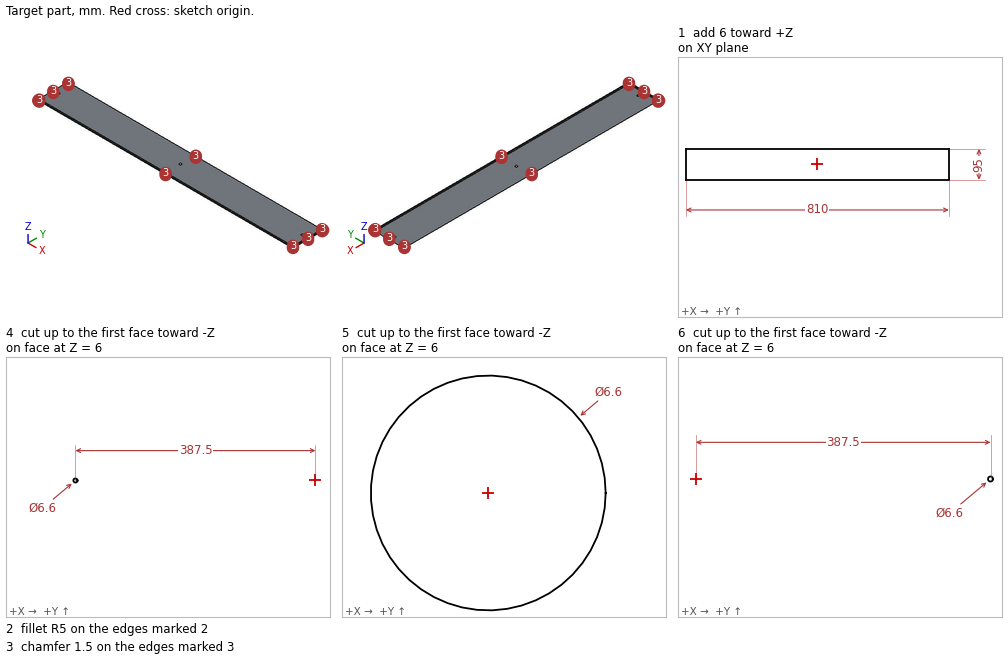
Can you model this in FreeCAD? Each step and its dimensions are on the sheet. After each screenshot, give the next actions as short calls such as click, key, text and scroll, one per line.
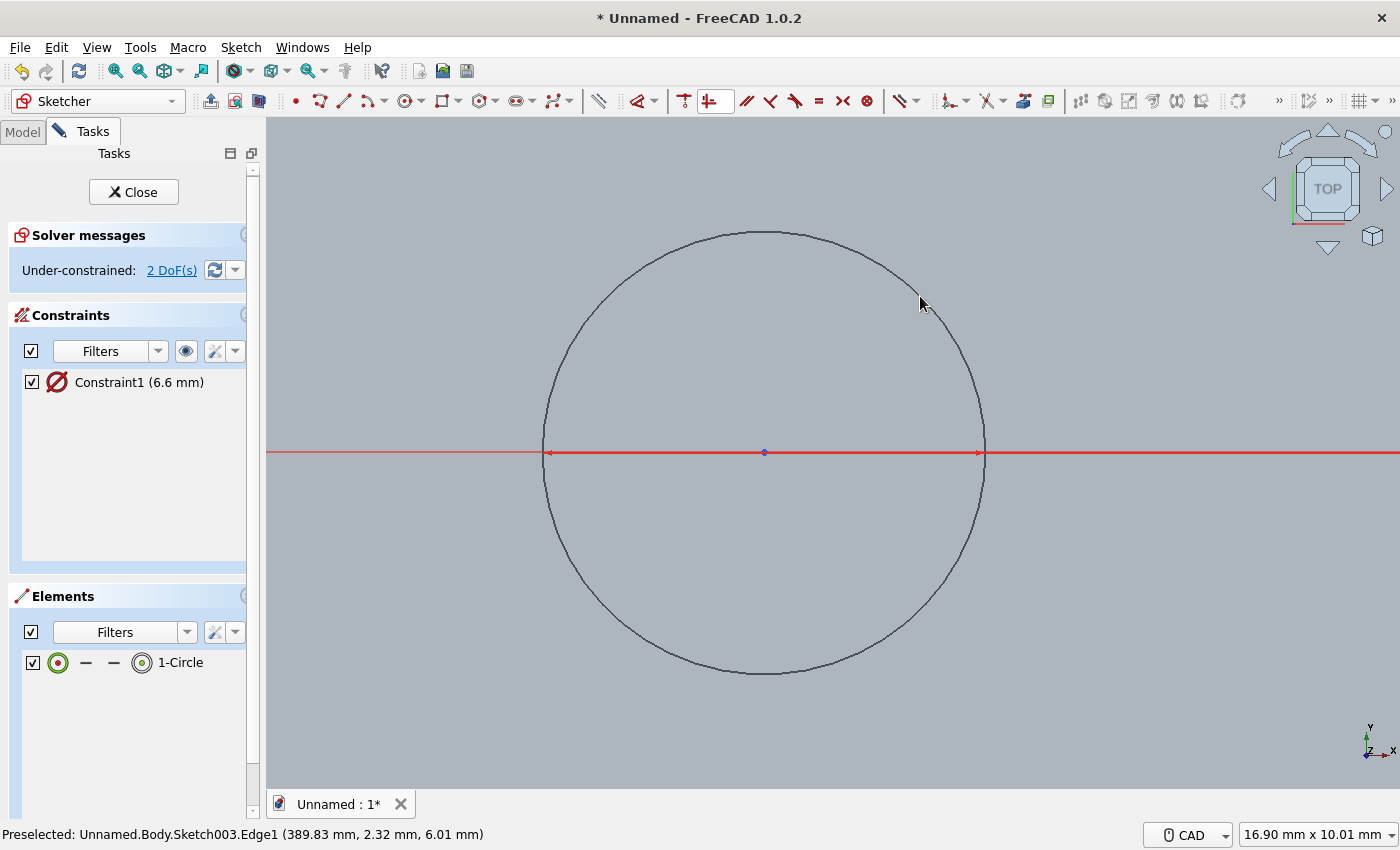
click(764, 453)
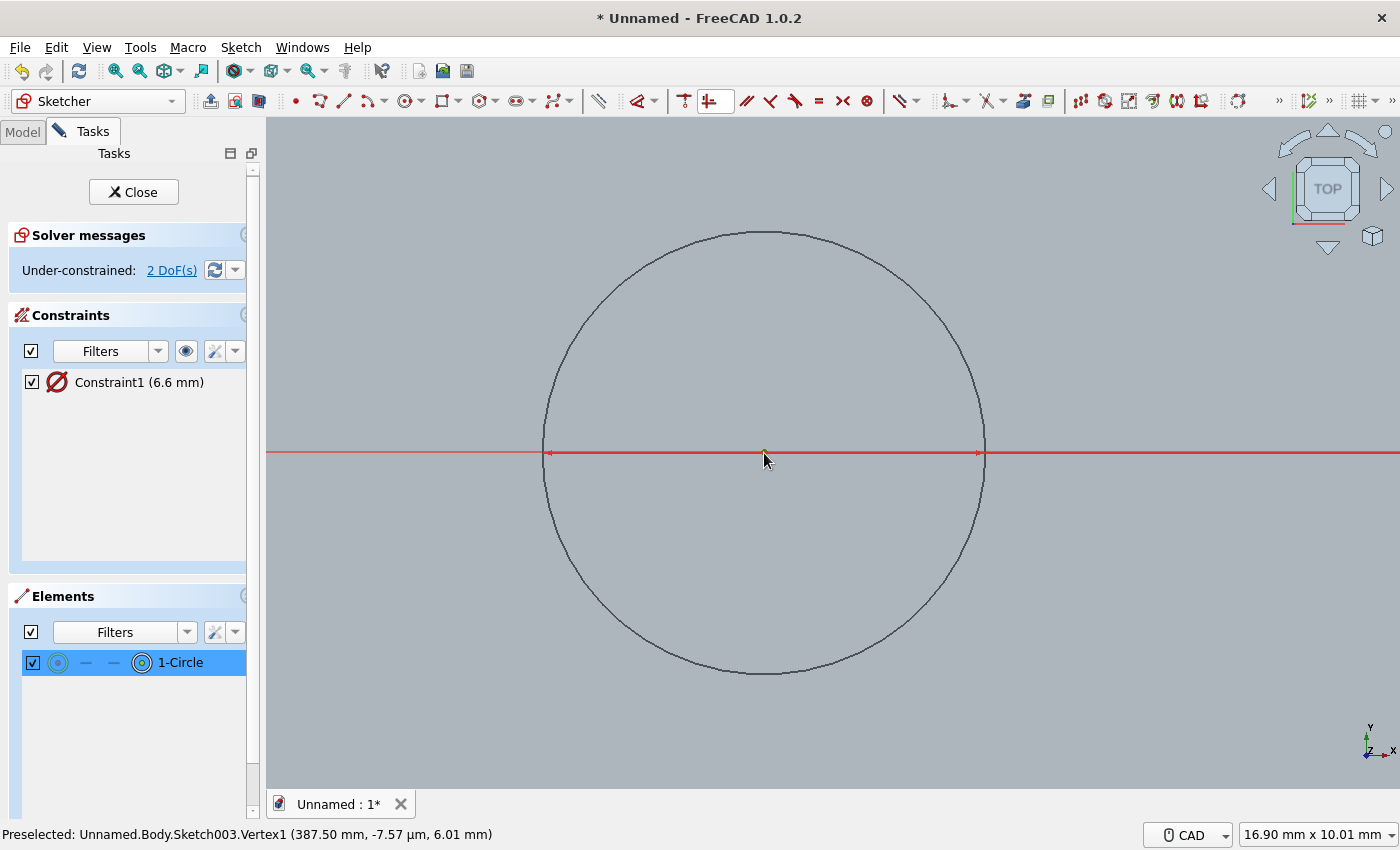
click(361, 452)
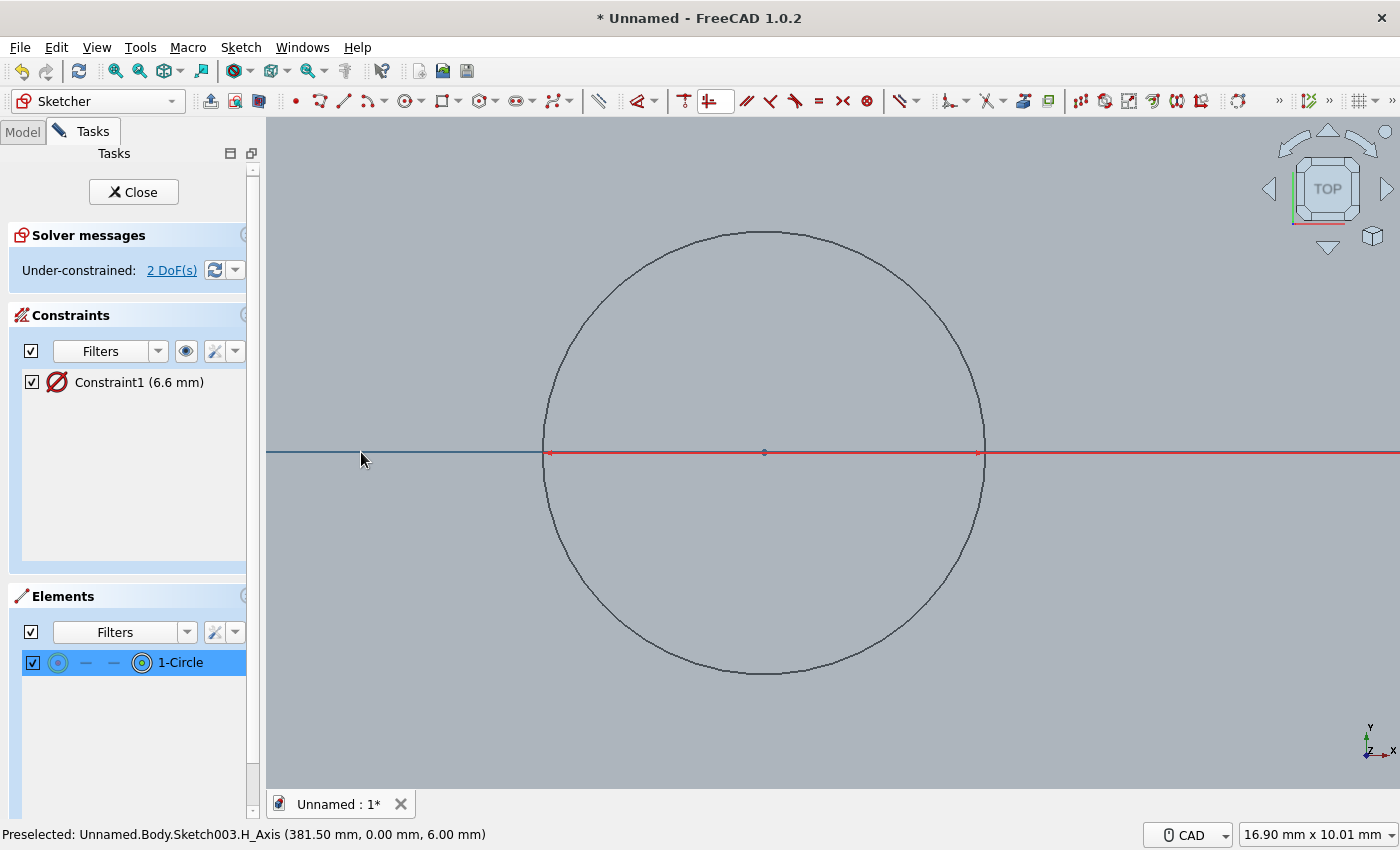
key(c)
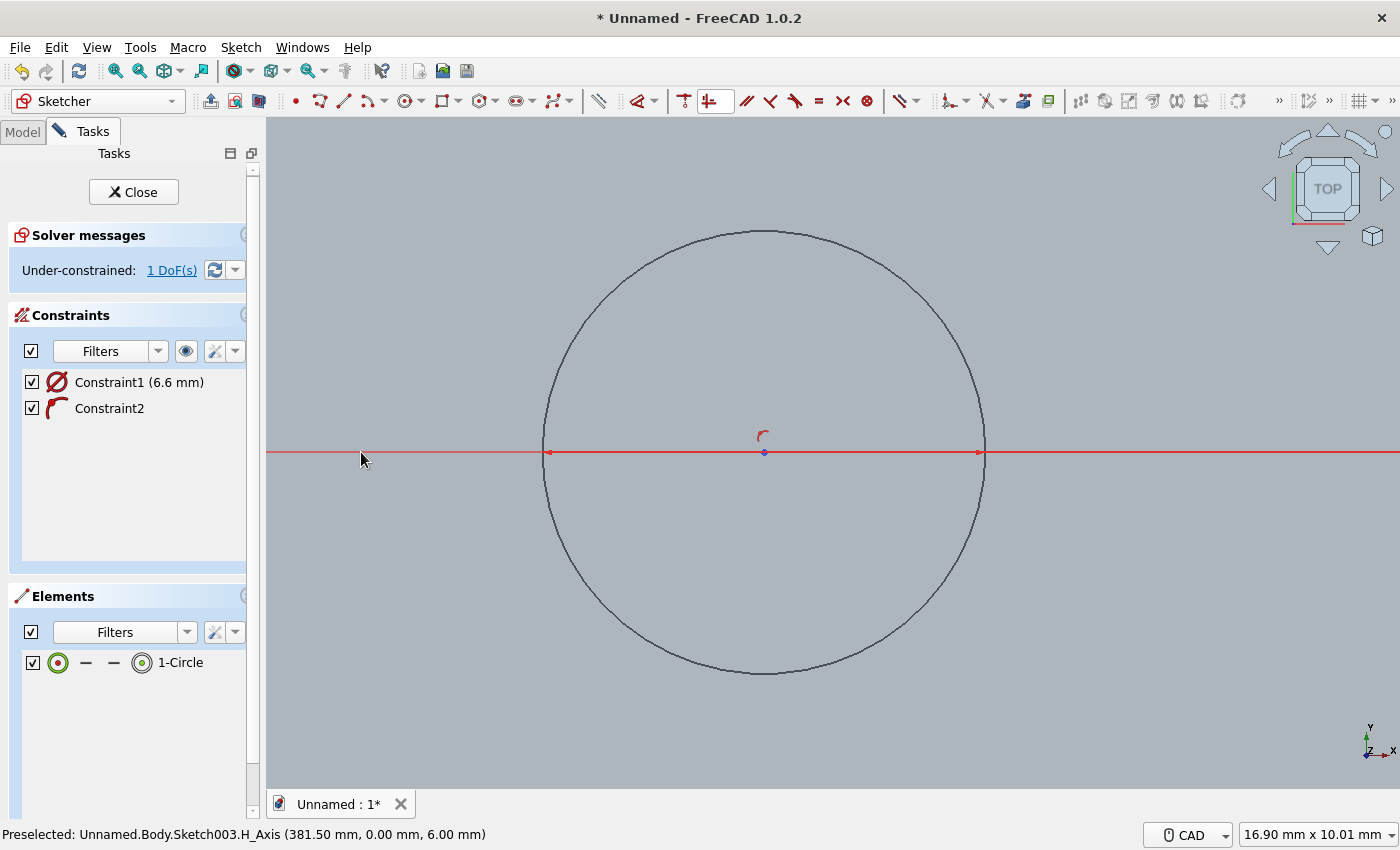
key(d)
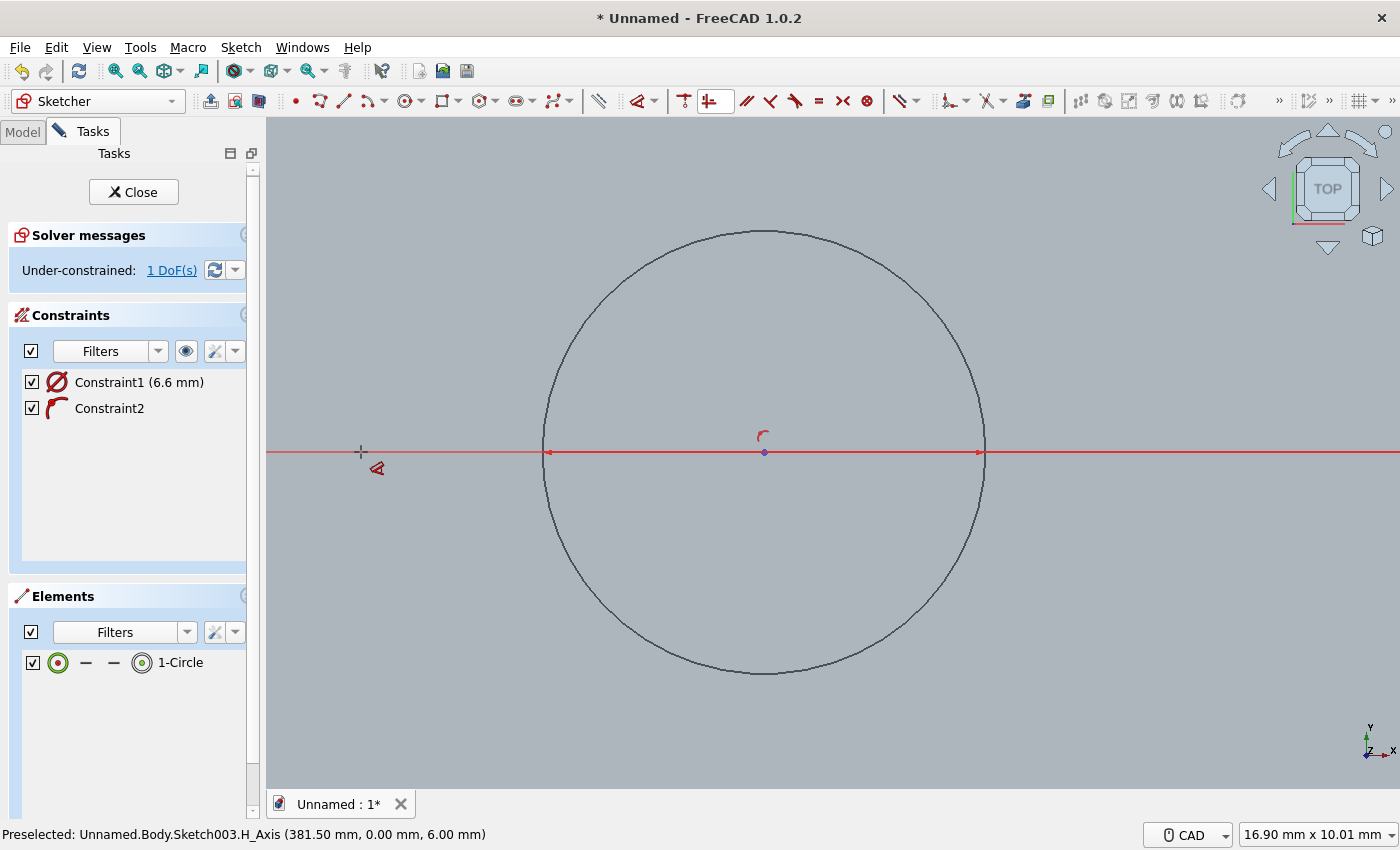
click(764, 452)
click(529, 486)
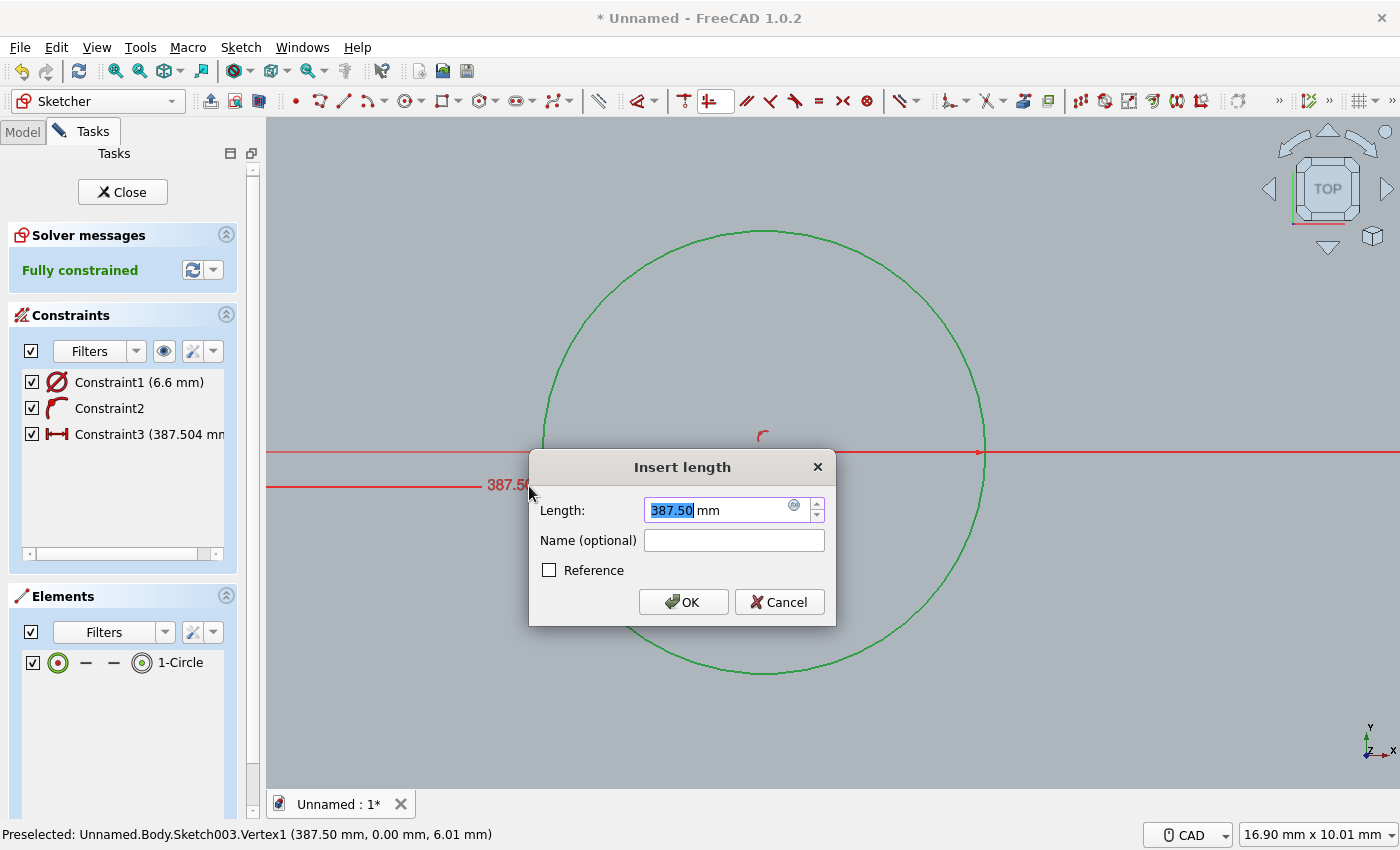
text(387.5)
key(Return)
key(Escape)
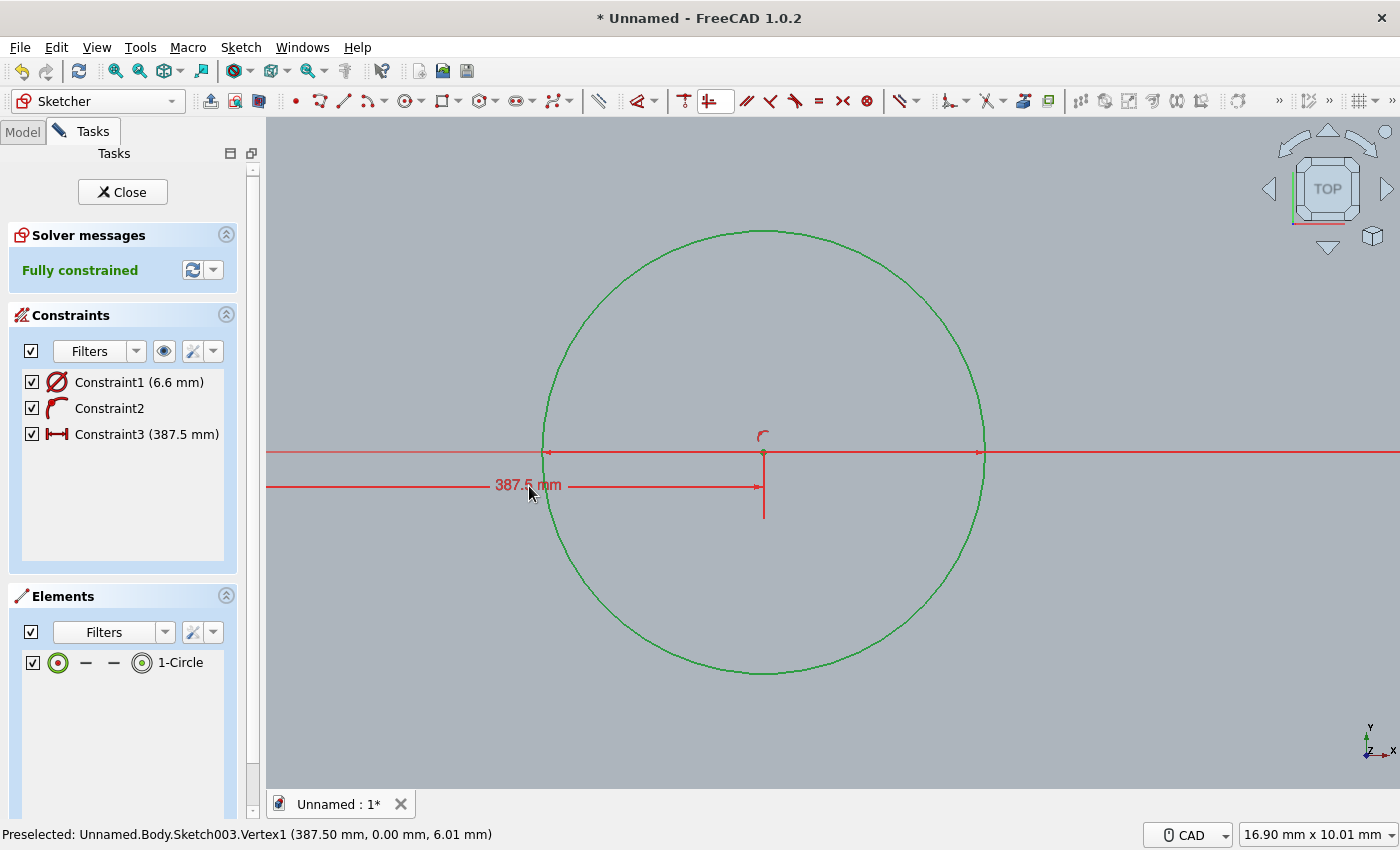
click(123, 192)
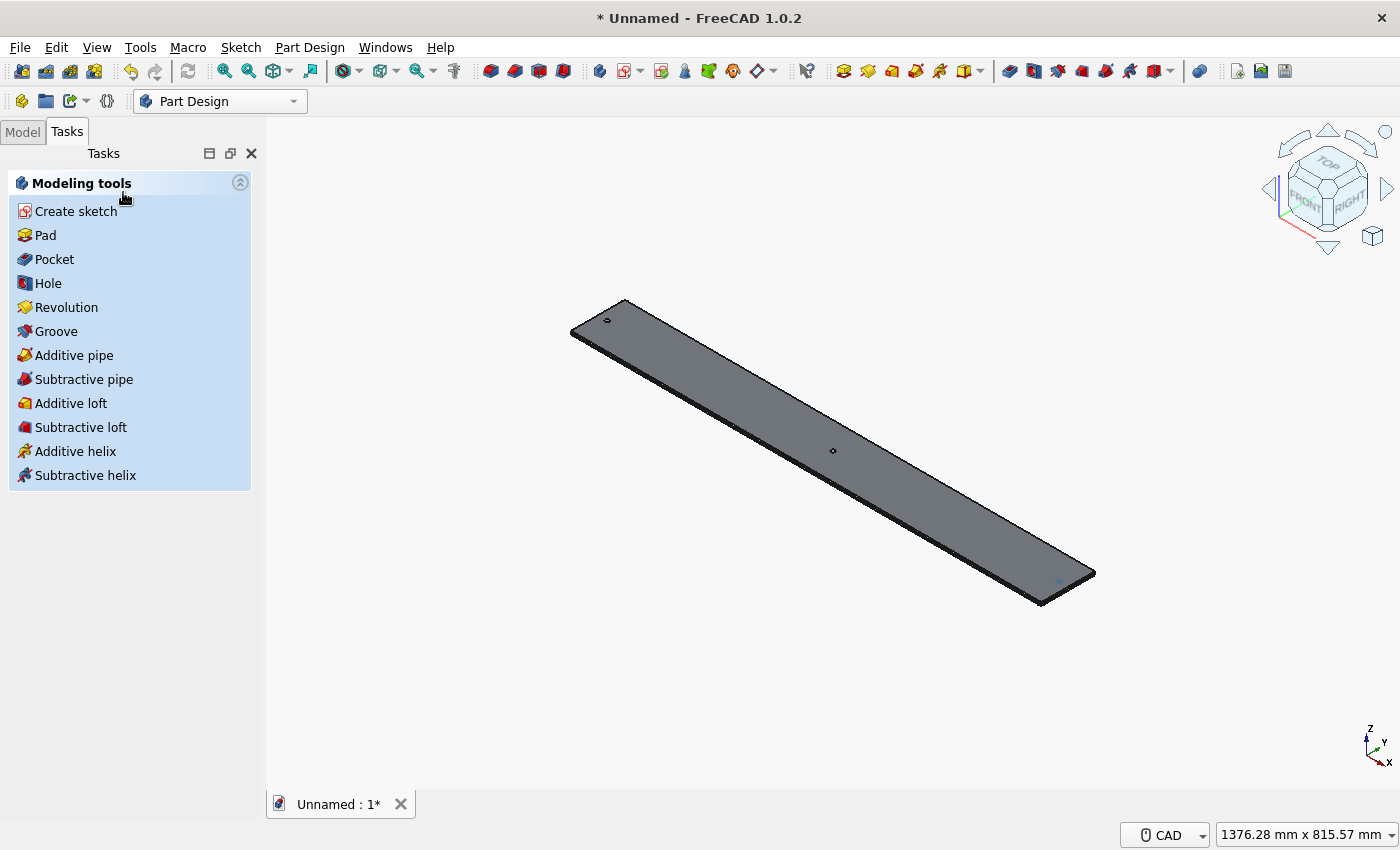
click(1010, 72)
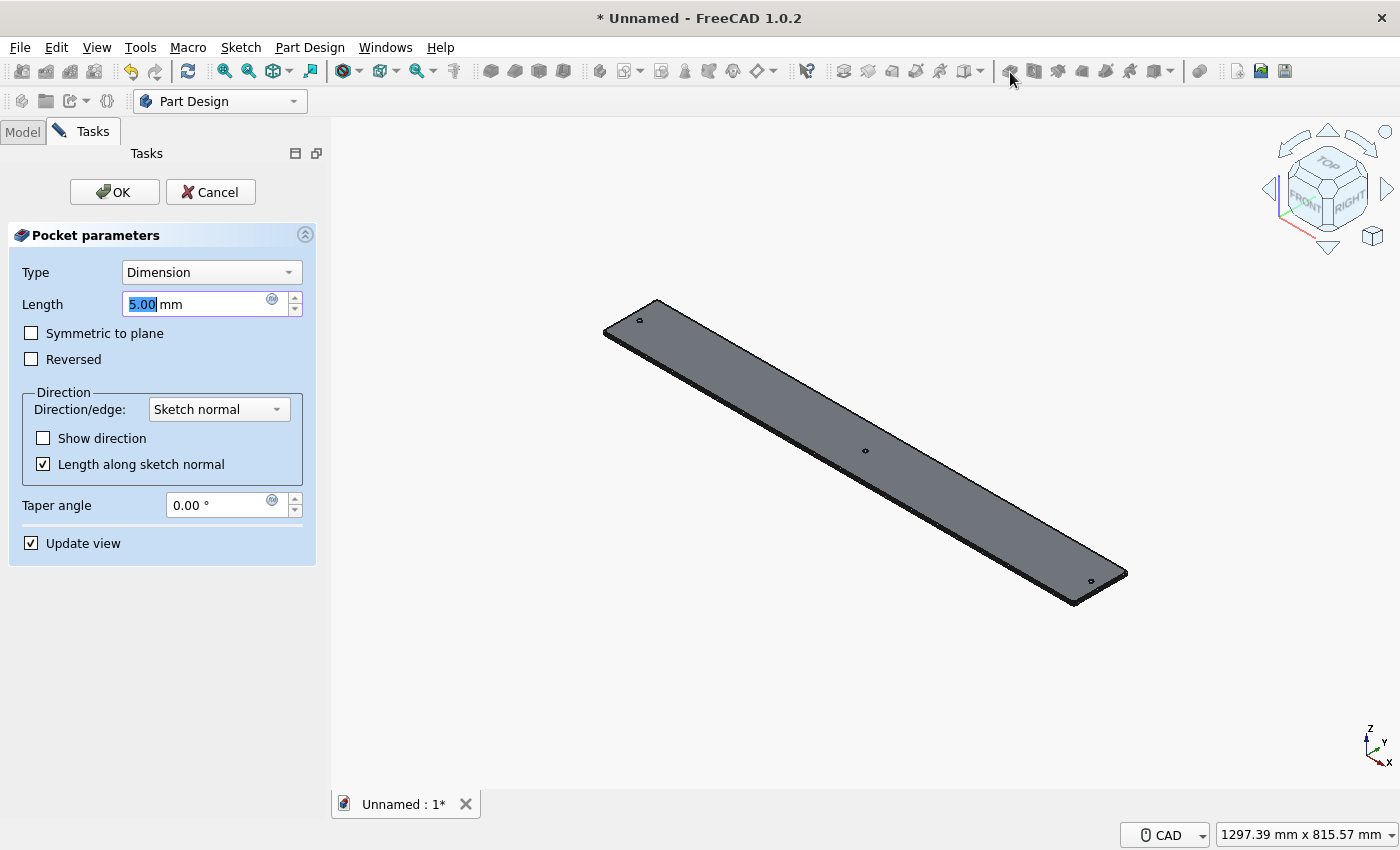
click(212, 272)